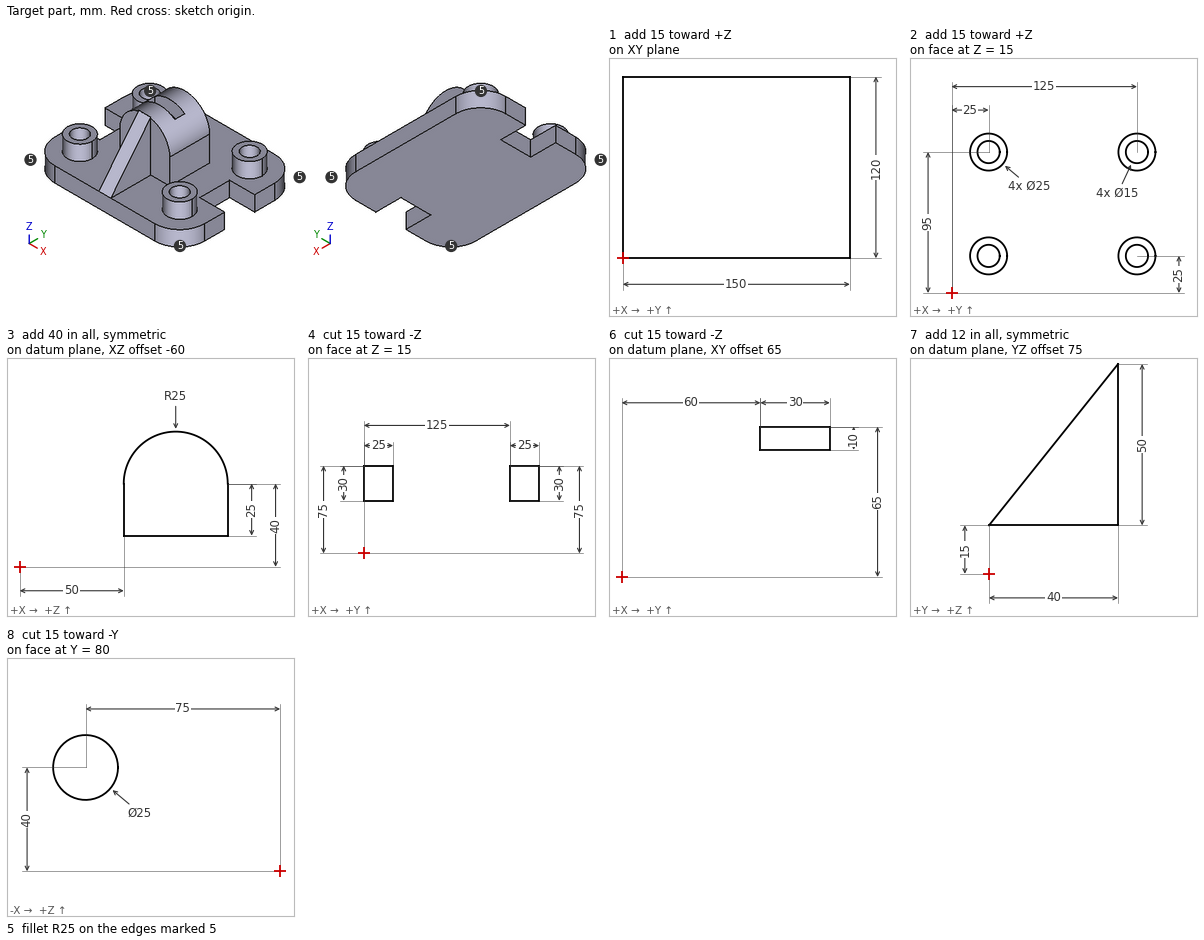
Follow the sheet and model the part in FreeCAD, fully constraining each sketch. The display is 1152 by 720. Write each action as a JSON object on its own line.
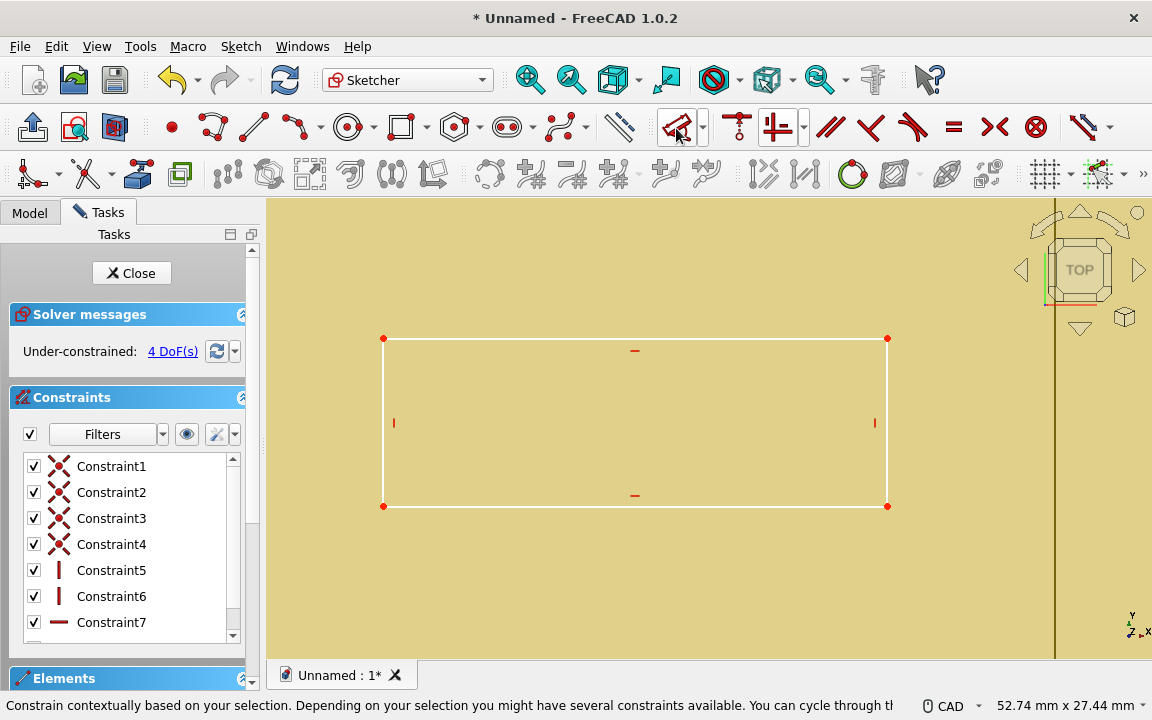
{"action": "left_click", "coordinate": [383, 389]}
{"action": "left_click", "coordinate": [349, 423]}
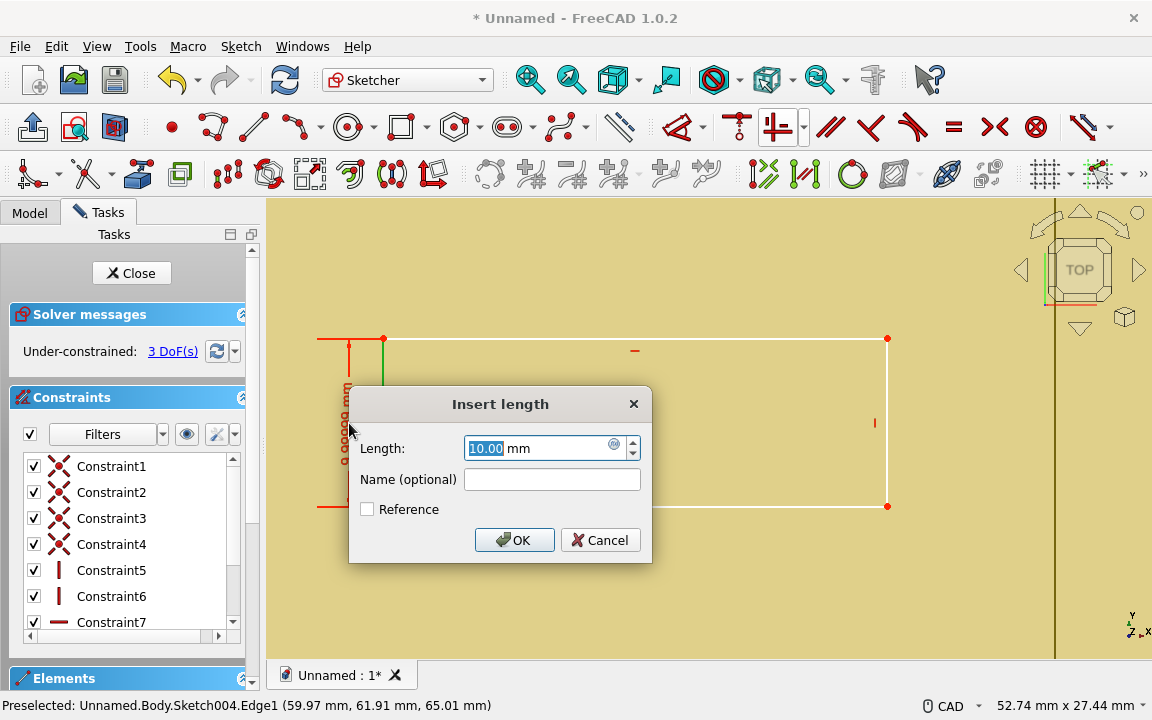
{"action": "type", "text": "10"}
{"action": "key", "text": "Return"}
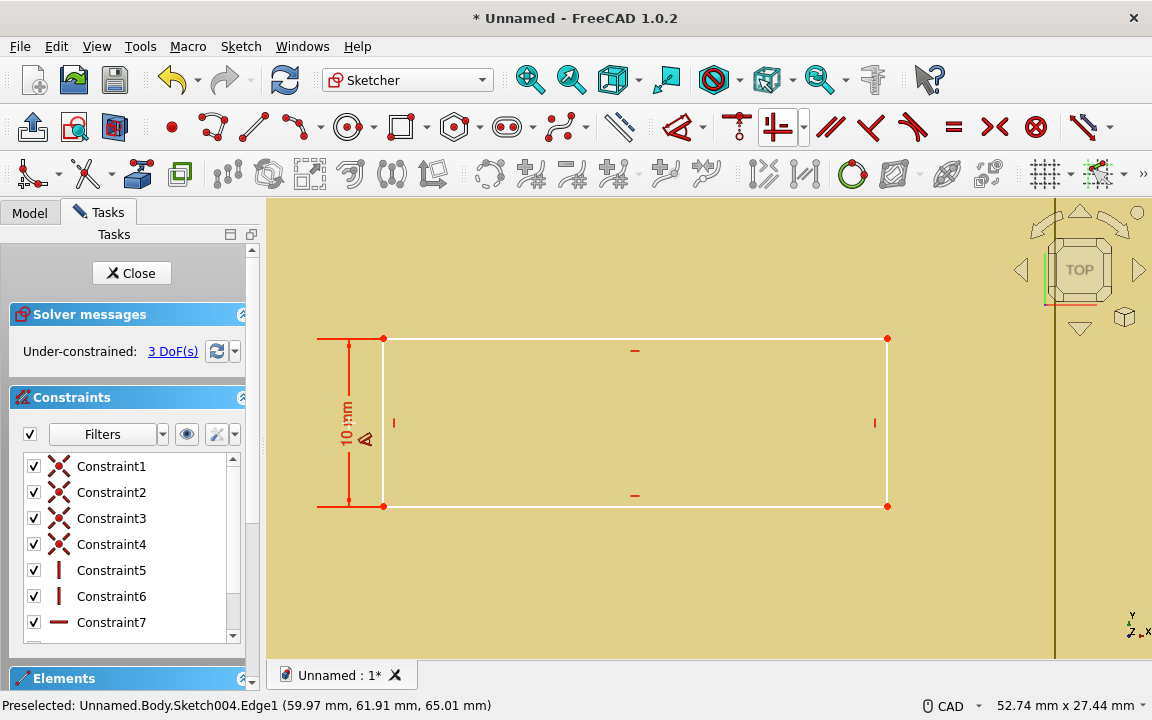
{"action": "left_click", "coordinate": [534, 507]}
{"action": "left_click", "coordinate": [635, 541]}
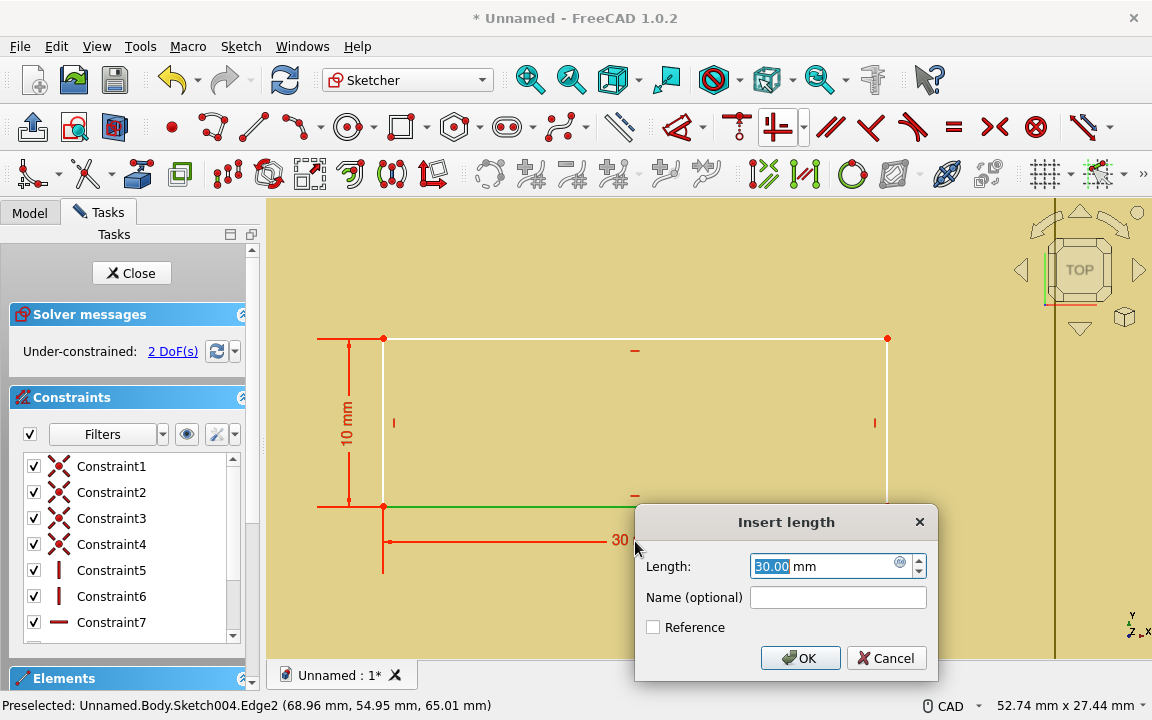
{"action": "type", "text": "30"}
{"action": "key", "text": "Return"}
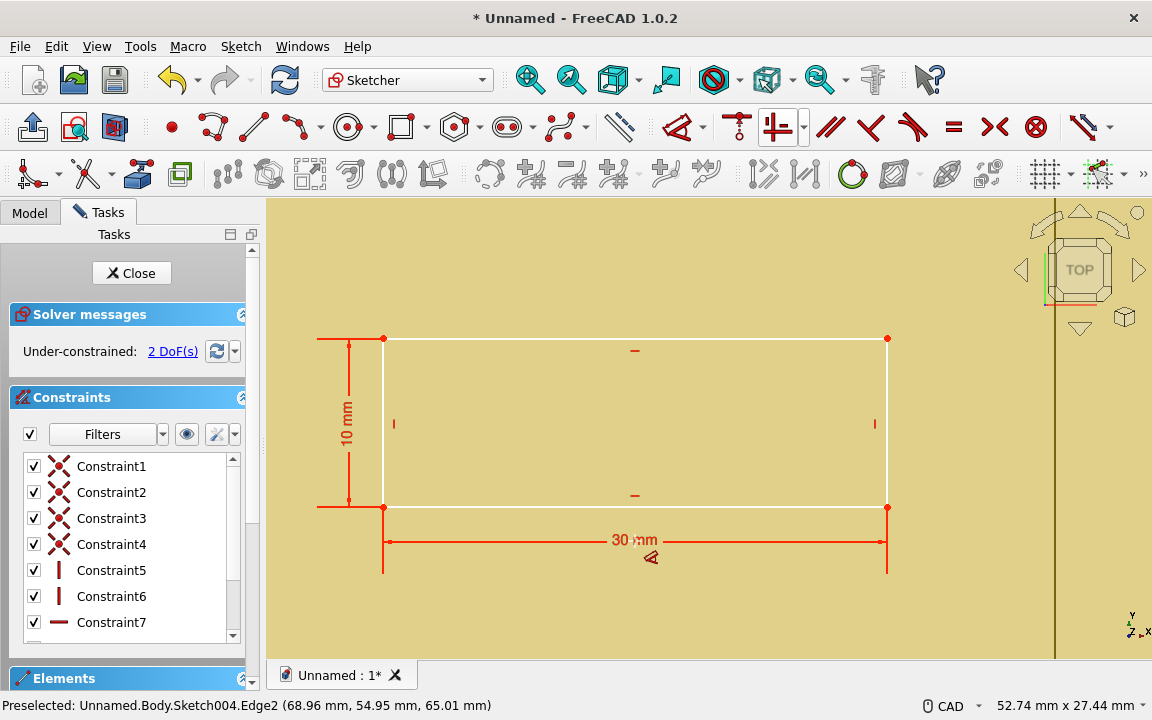
{"action": "left_click", "coordinate": [383, 339]}
{"action": "left_click", "coordinate": [339, 305]}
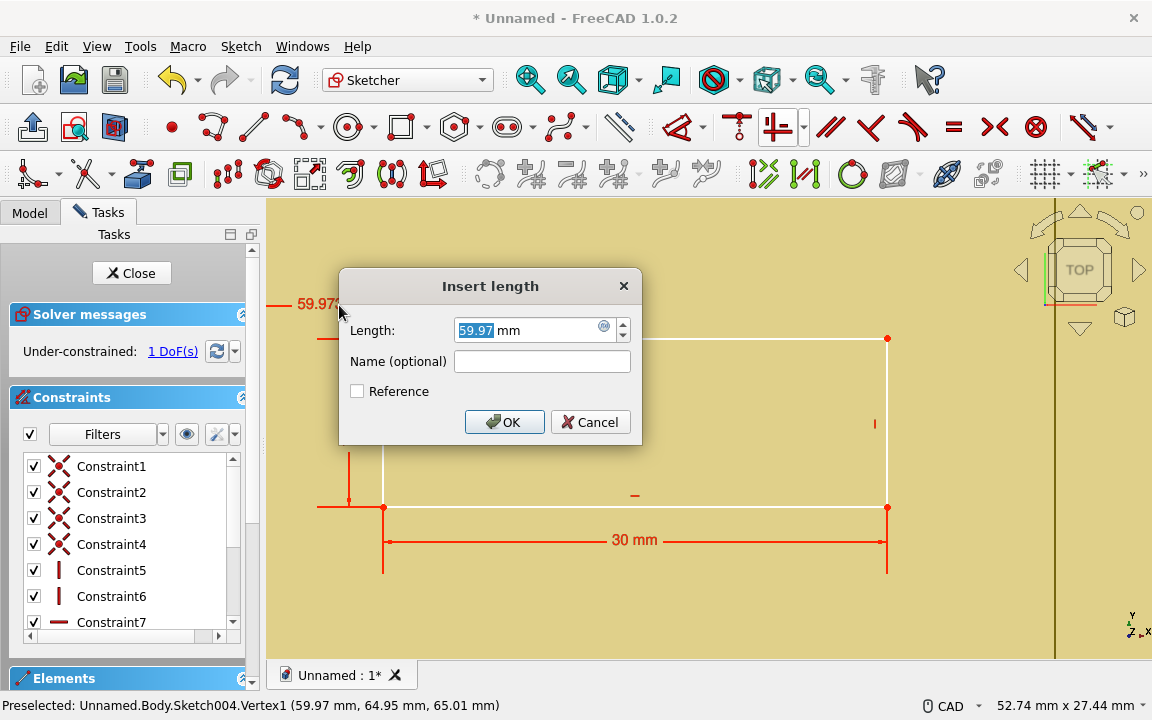
{"action": "type", "text": "60"}
{"action": "key", "text": "Return"}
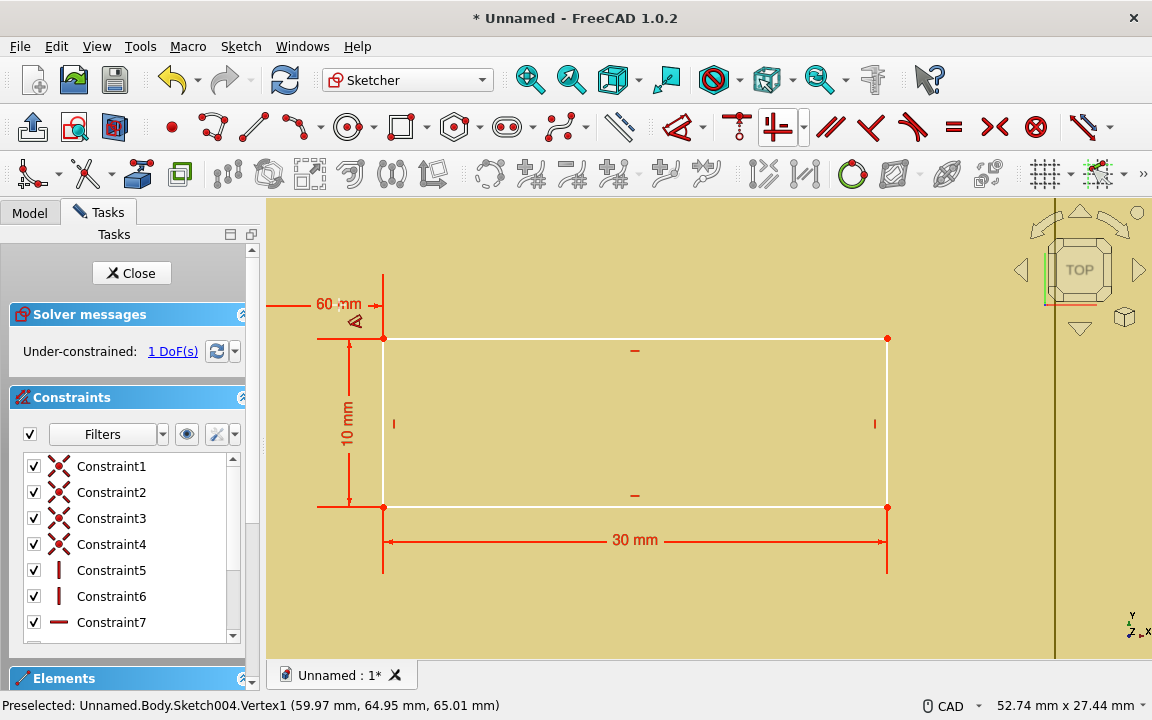
{"action": "left_click", "coordinate": [383, 339]}
{"action": "left_click", "coordinate": [417, 485]}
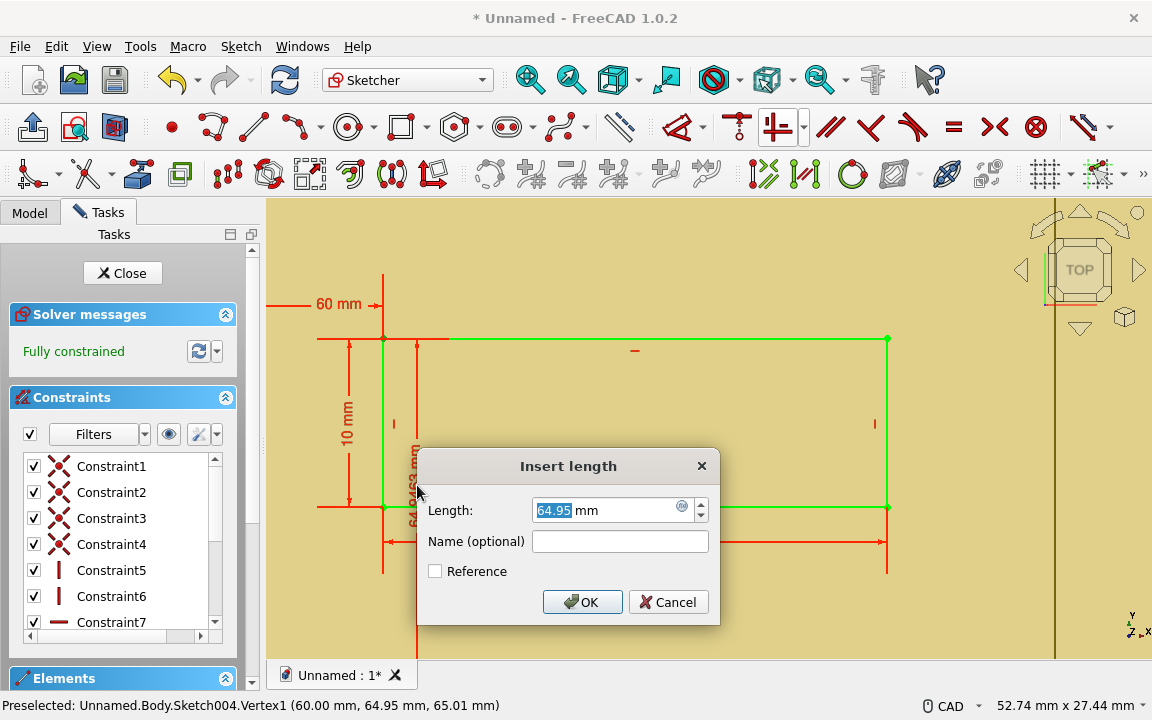
{"action": "type", "text": "65"}
{"action": "key", "text": "Return"}
{"action": "key", "text": "Escape"}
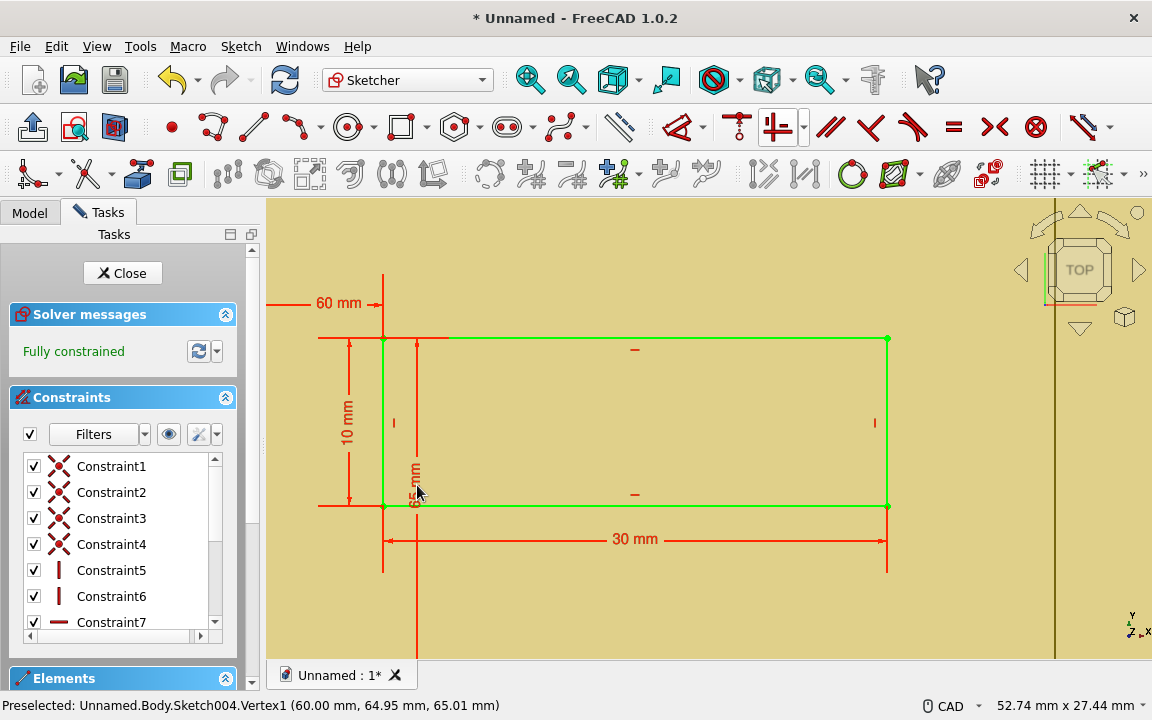
{"action": "left_click", "coordinate": [123, 273]}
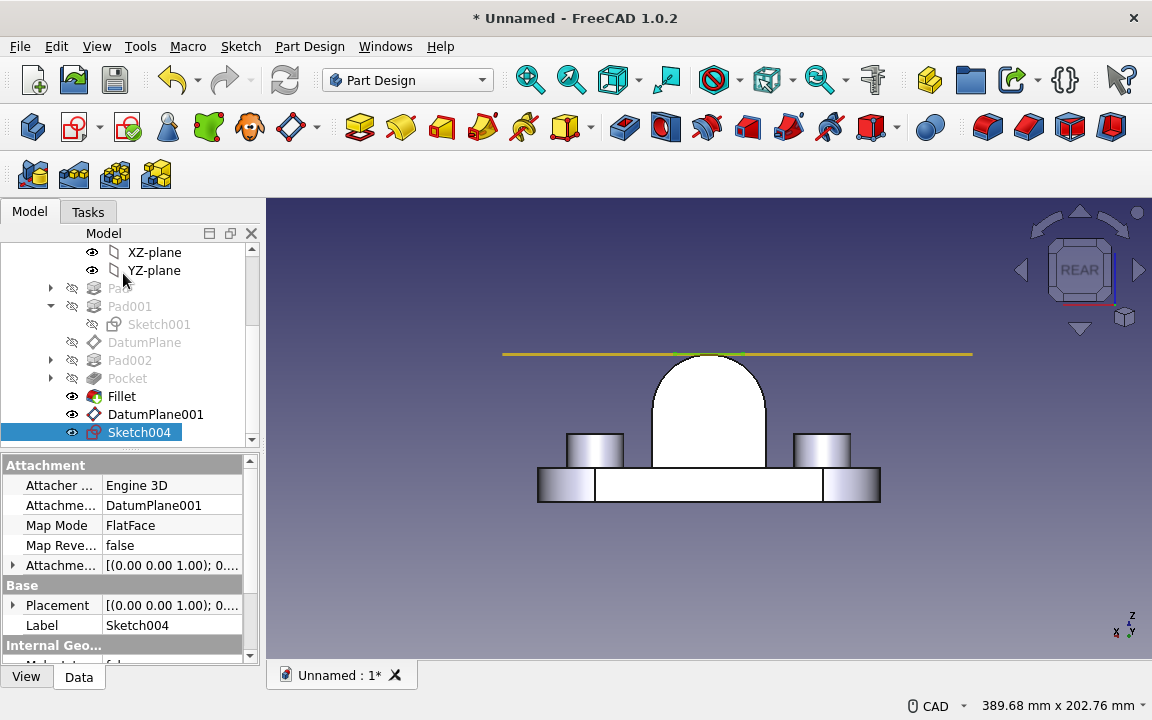
{"action": "left_click", "coordinate": [625, 128]}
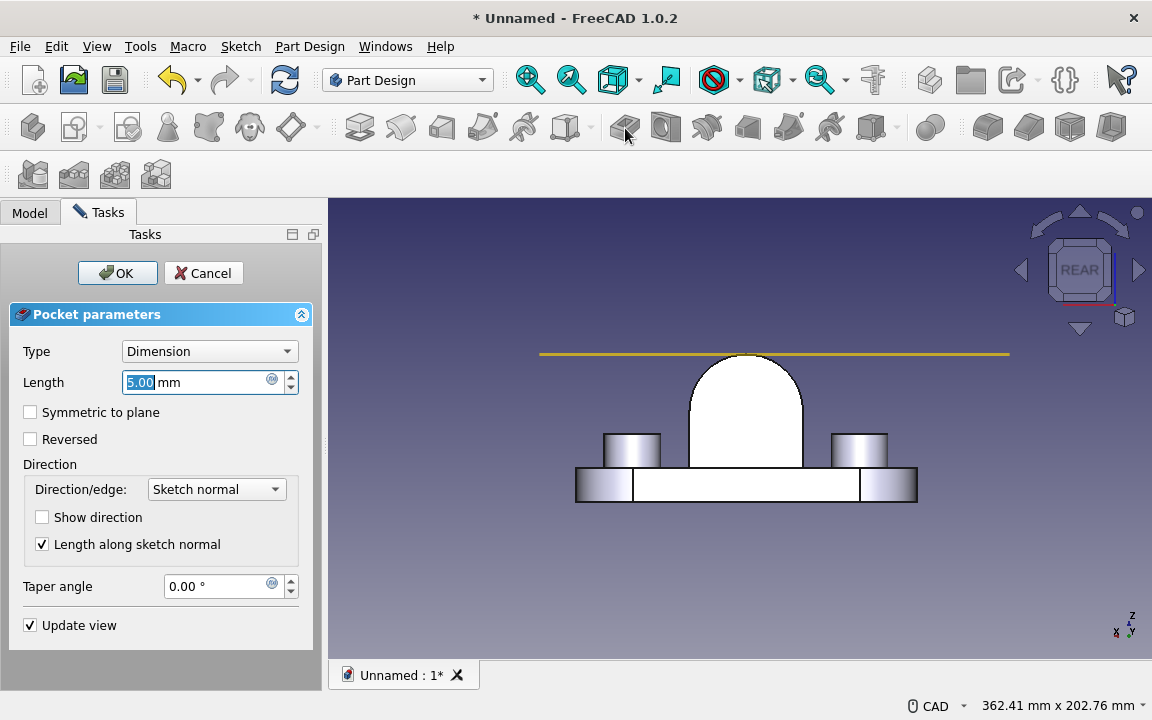
{"action": "type", "text": "15"}
{"action": "key", "text": "Tab"}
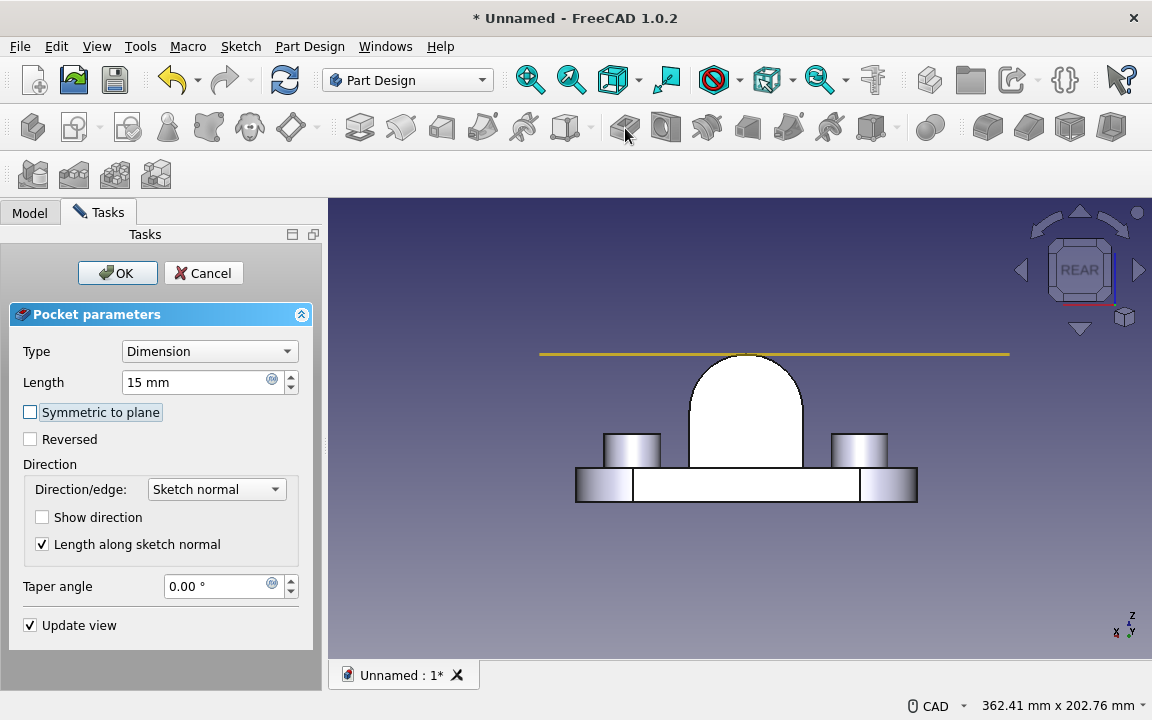
{"action": "left_click", "coordinate": [118, 273]}